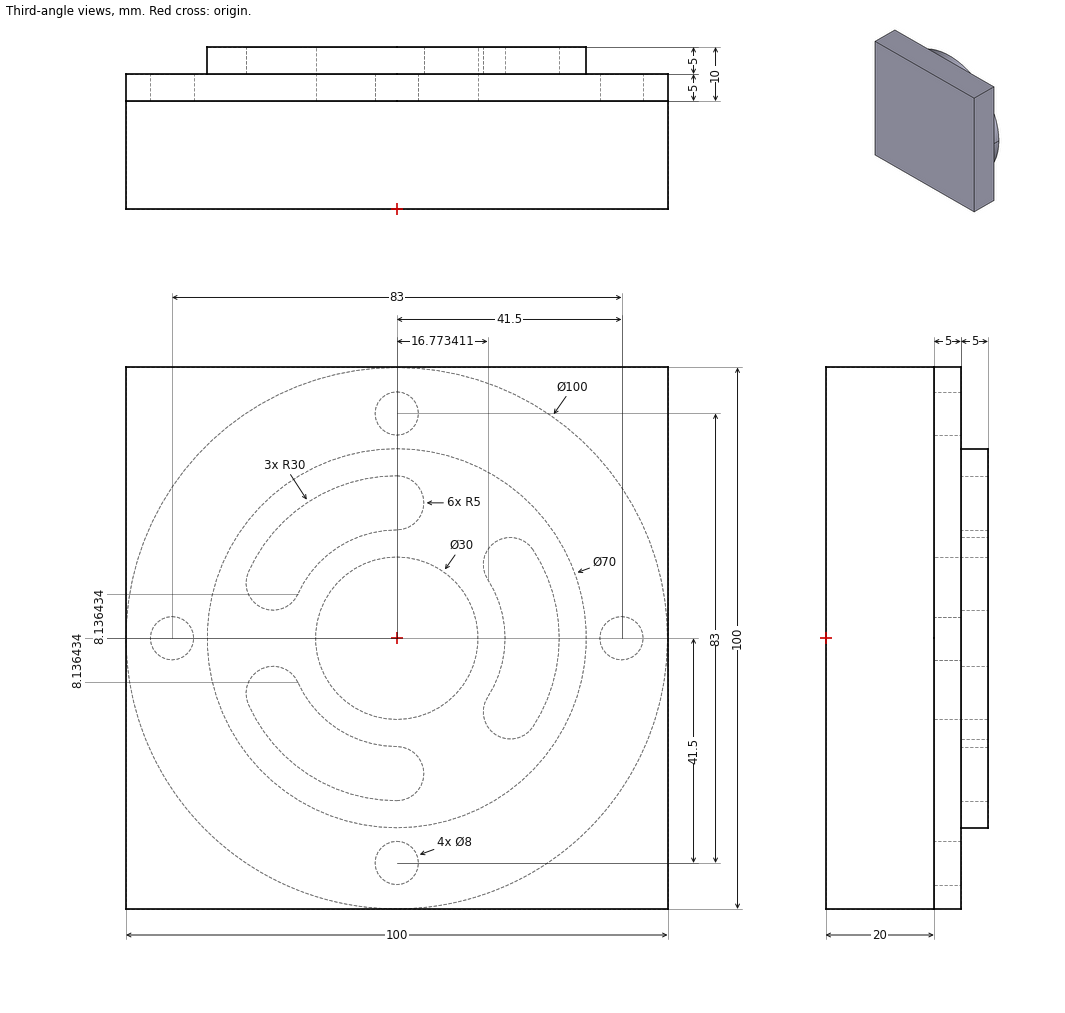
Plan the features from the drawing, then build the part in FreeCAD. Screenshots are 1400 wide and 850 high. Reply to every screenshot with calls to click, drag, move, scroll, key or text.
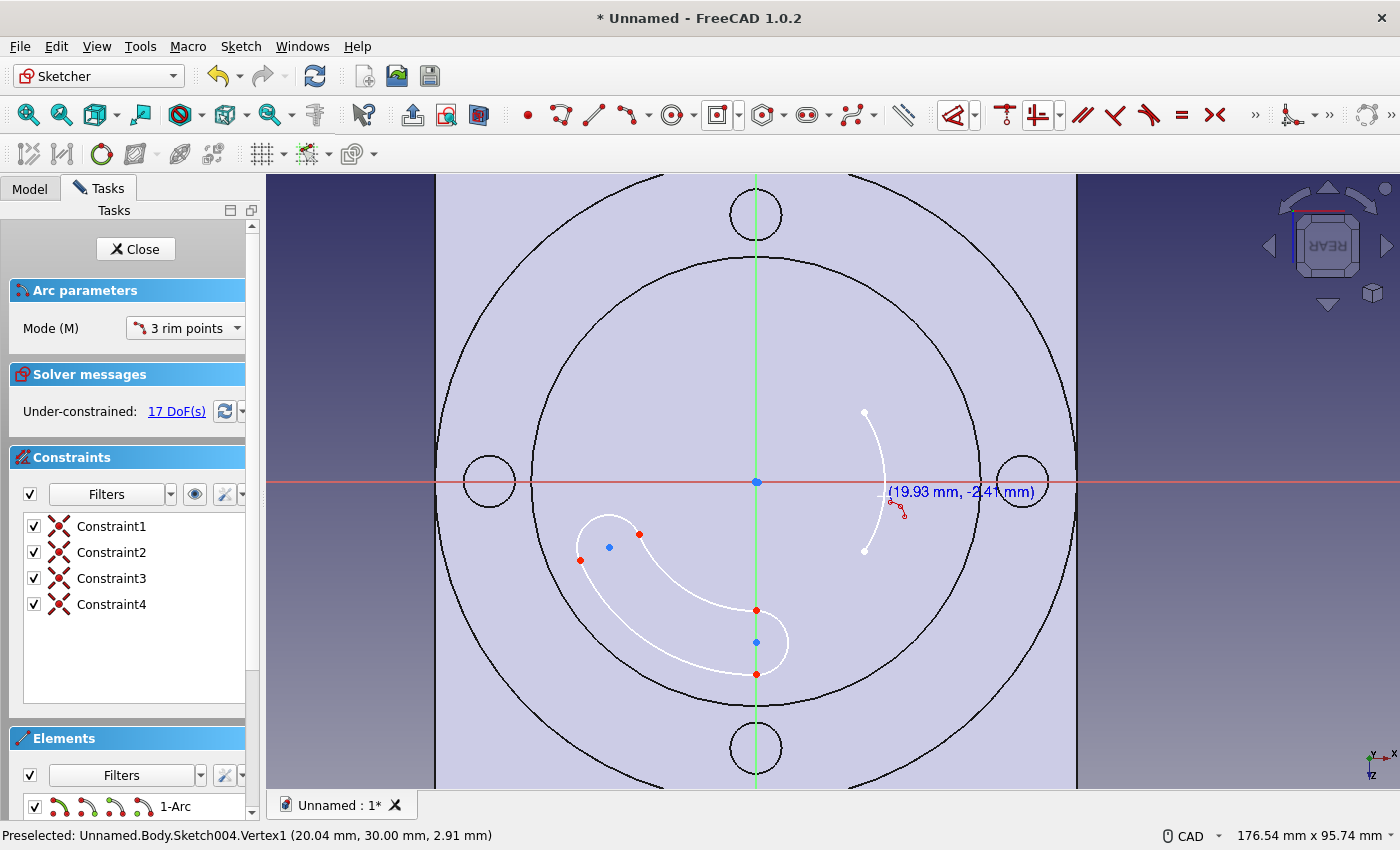
click(864, 552)
click(918, 586)
click(873, 596)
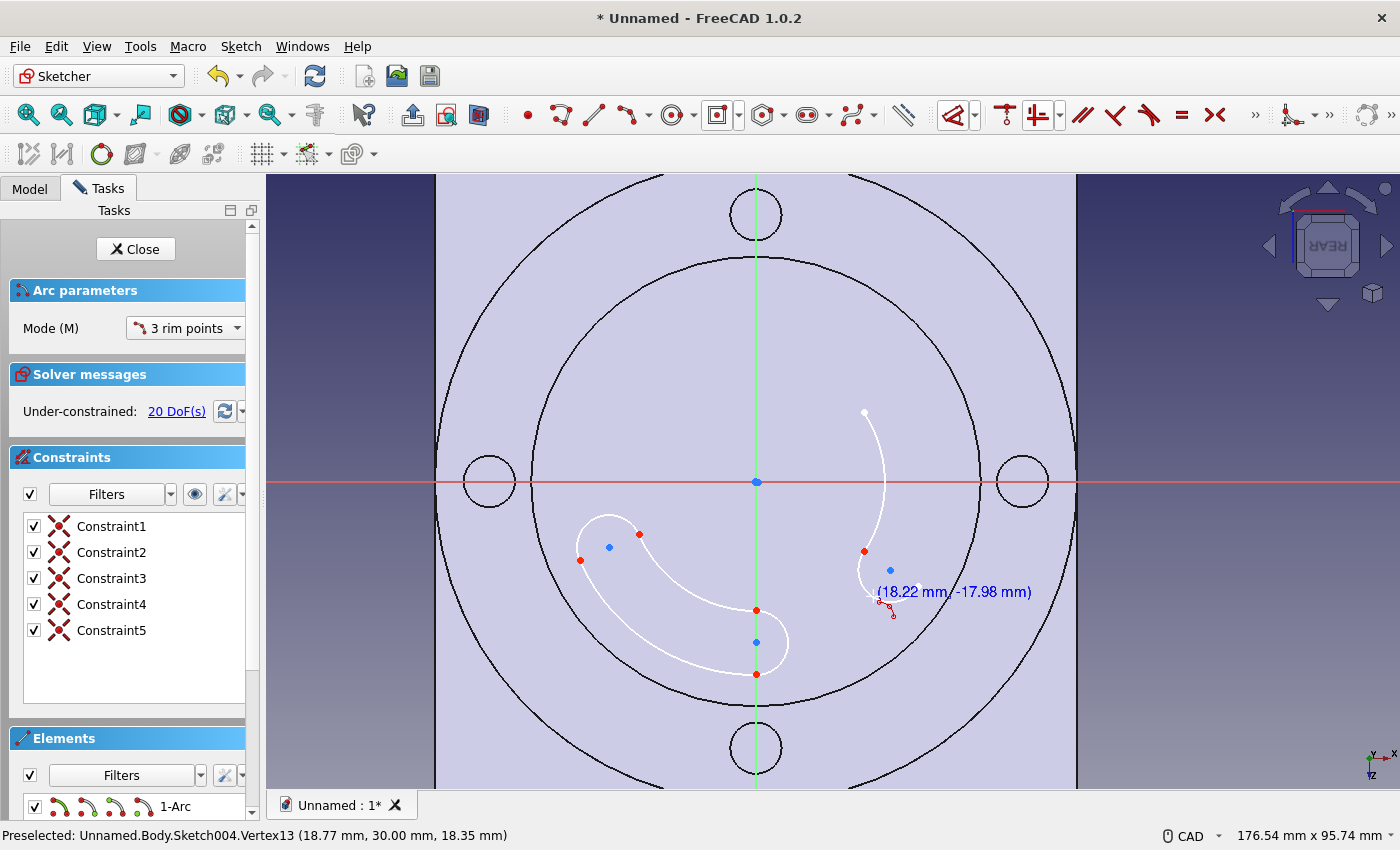
click(918, 587)
click(918, 377)
click(947, 504)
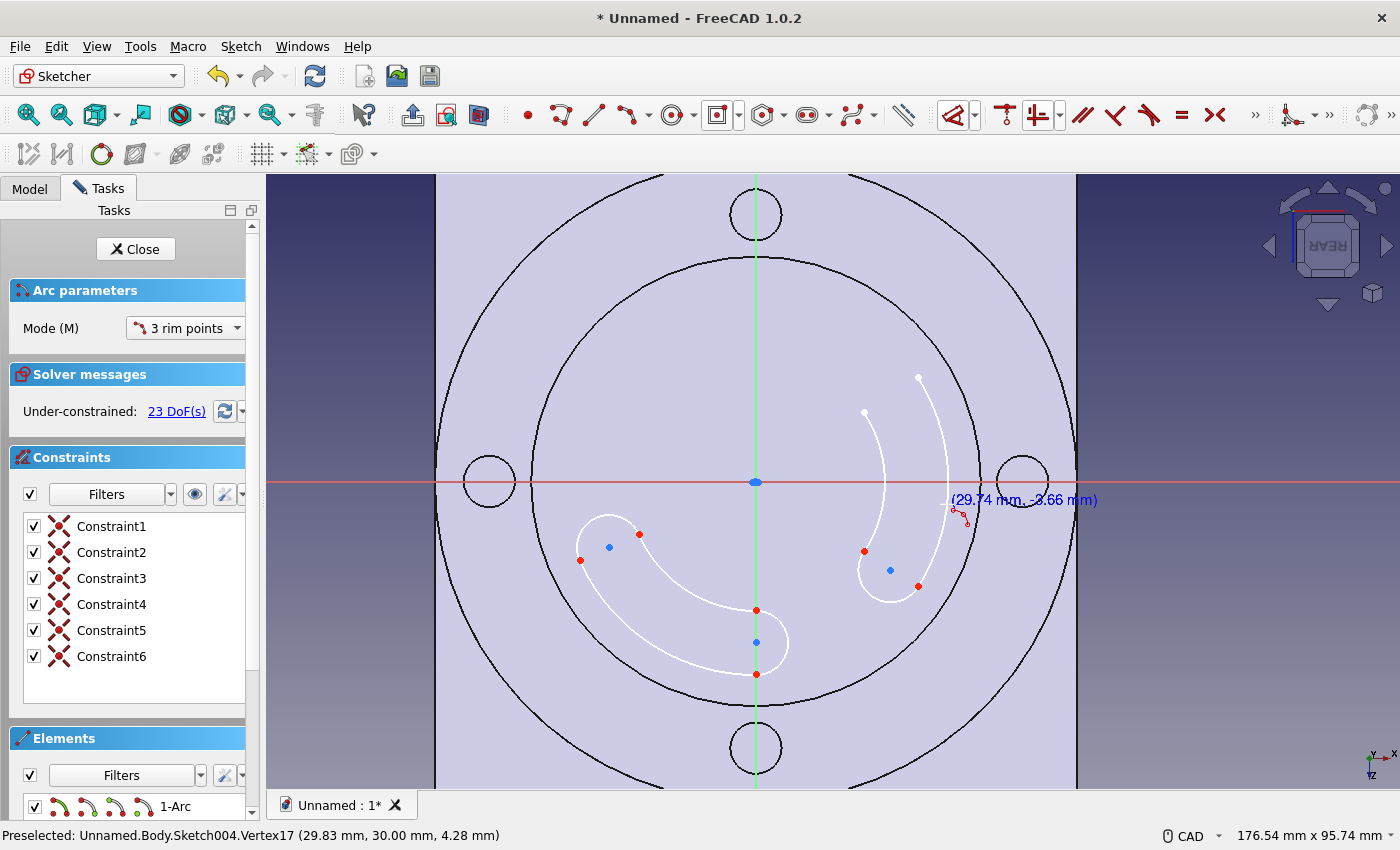
click(918, 378)
click(864, 413)
click(873, 367)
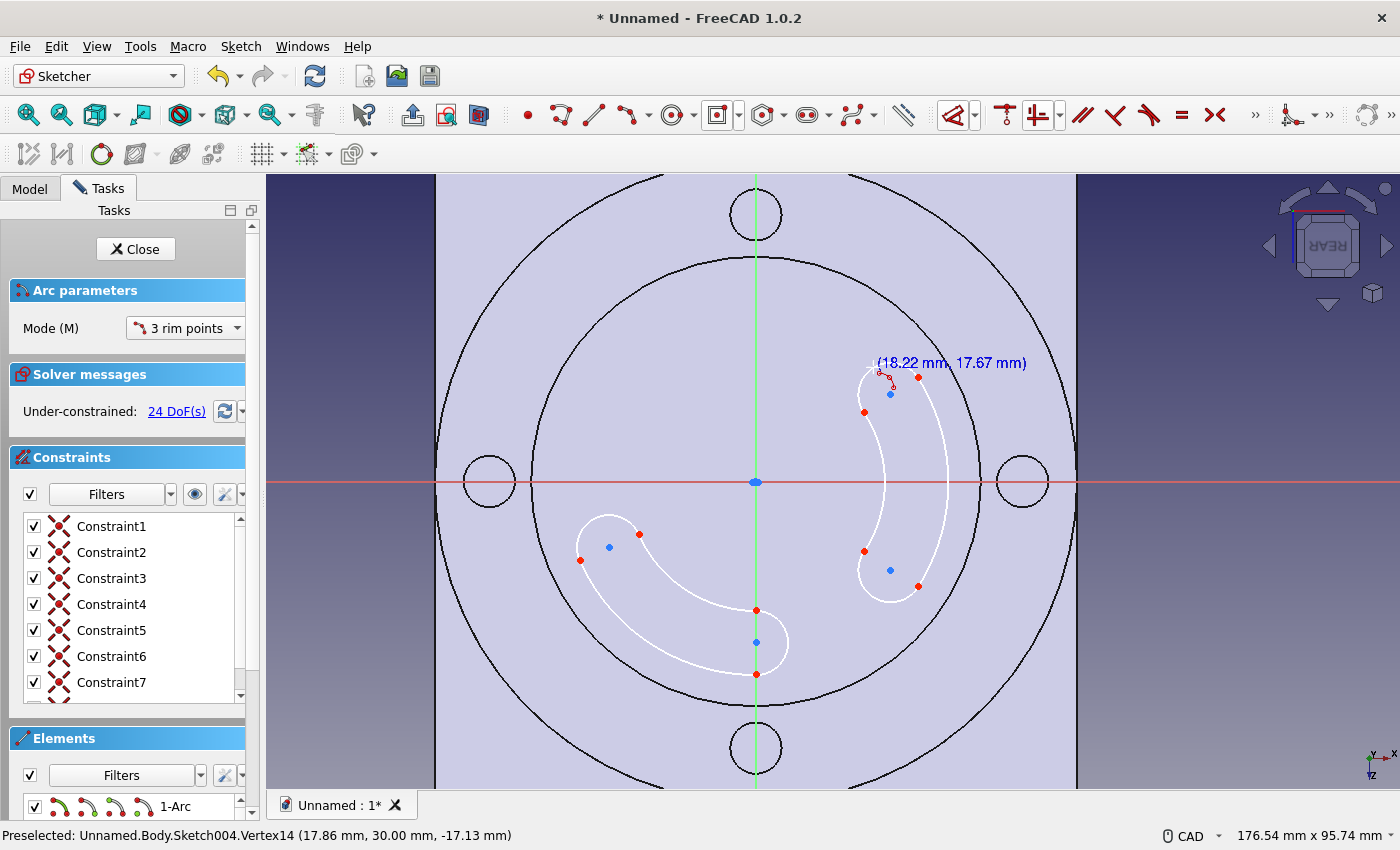
click(639, 429)
click(756, 353)
click(686, 374)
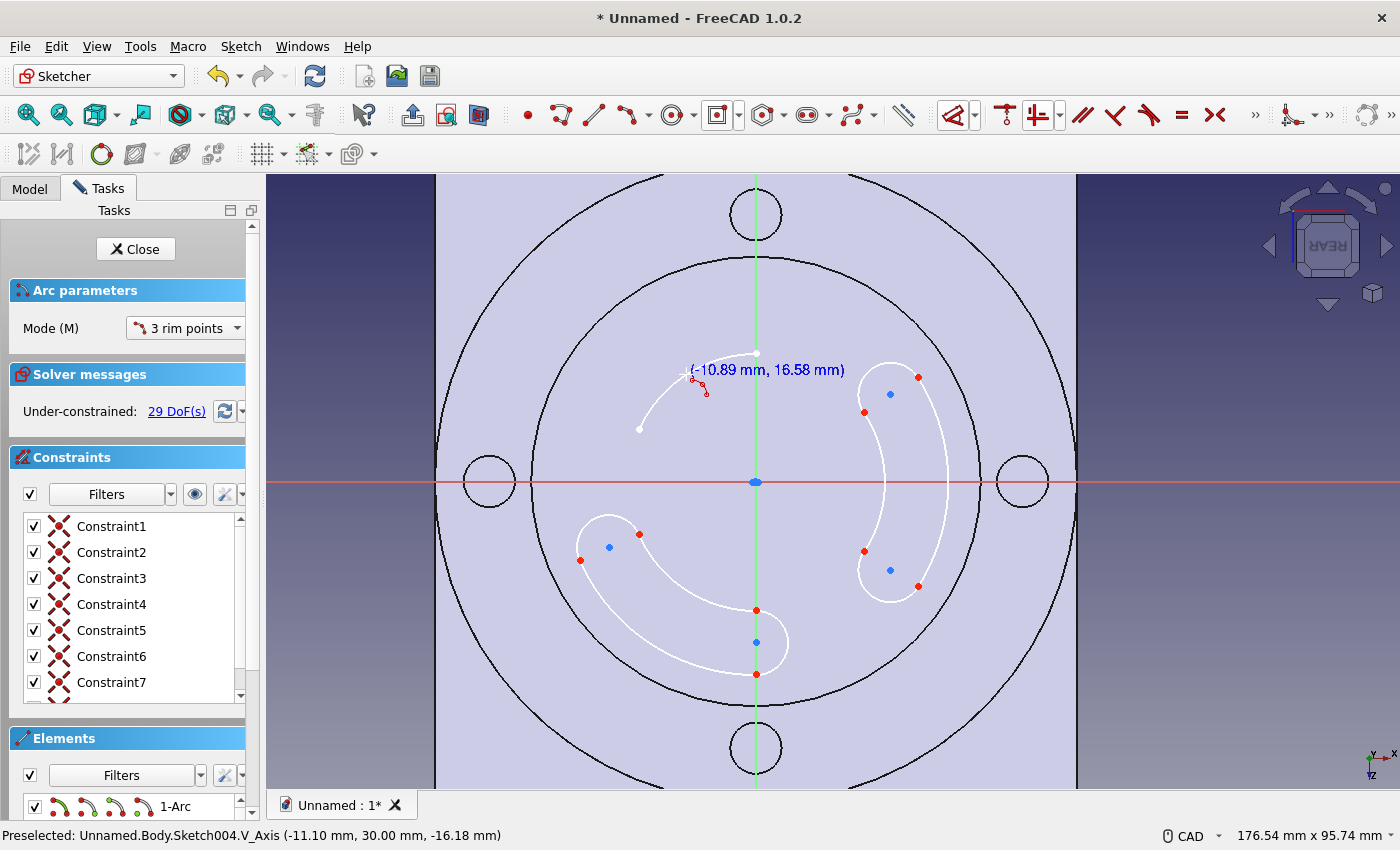
click(756, 354)
click(756, 289)
click(788, 321)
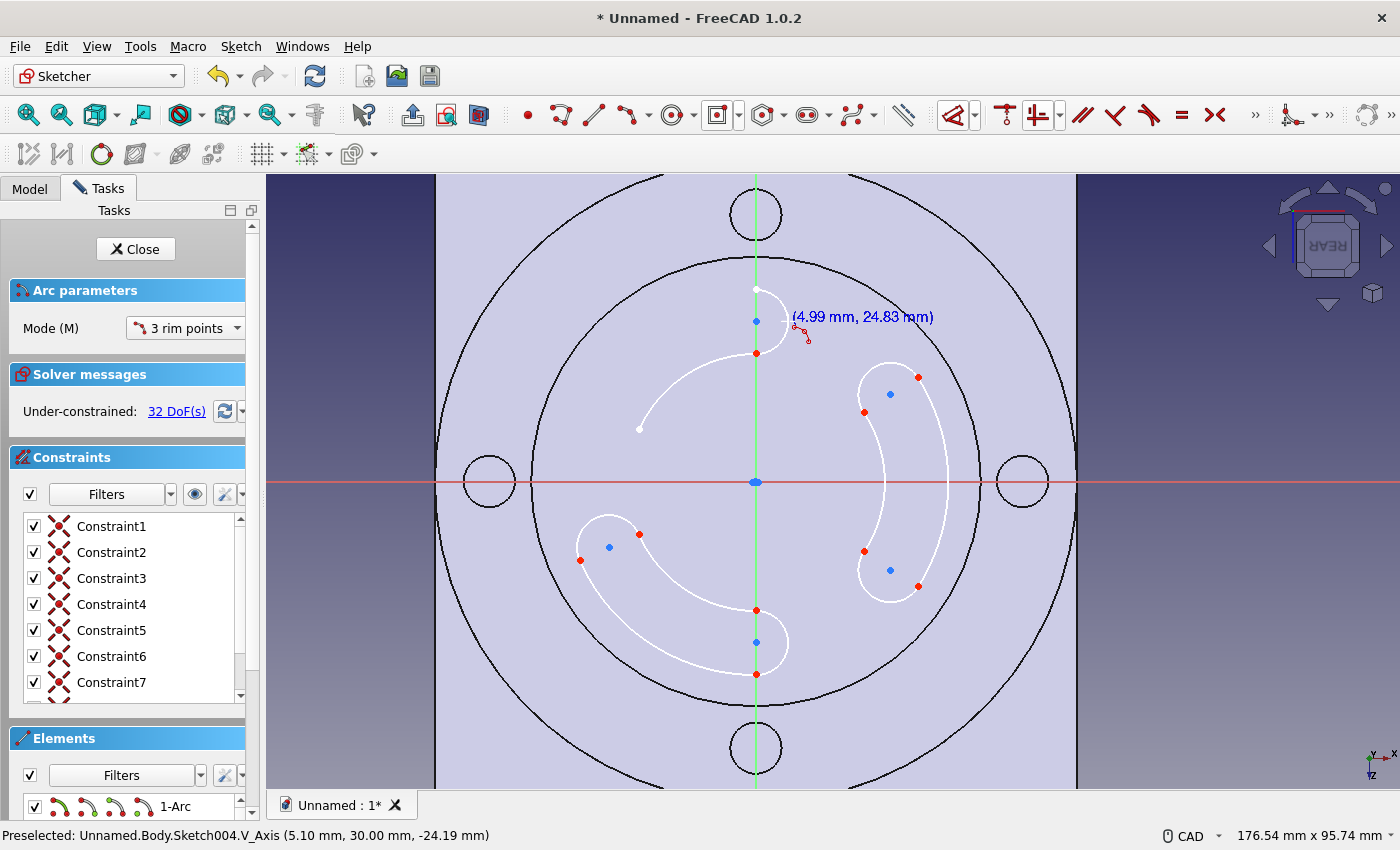
click(756, 290)
click(580, 403)
click(651, 320)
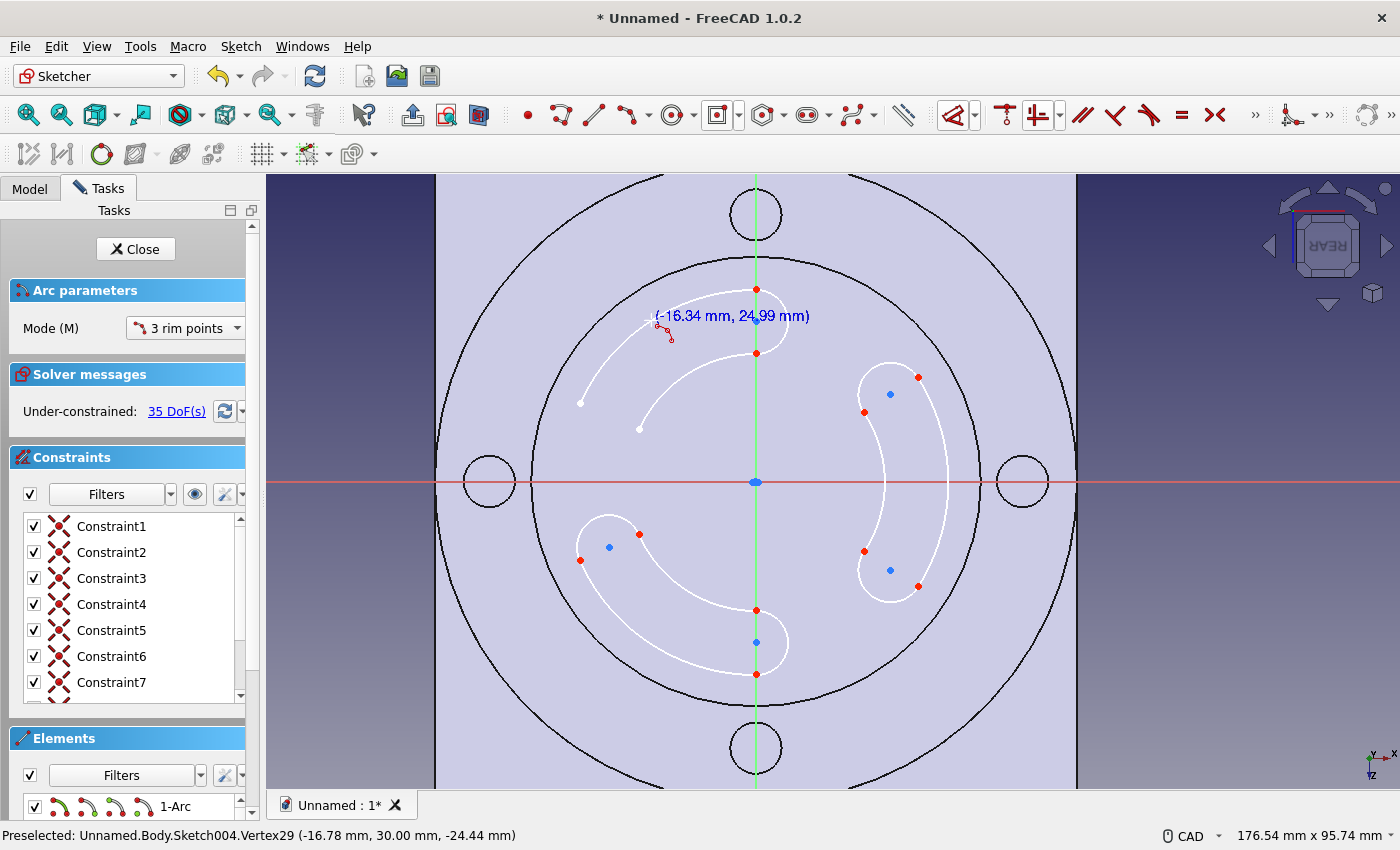
click(580, 404)
click(639, 430)
click(596, 446)
key(Escape)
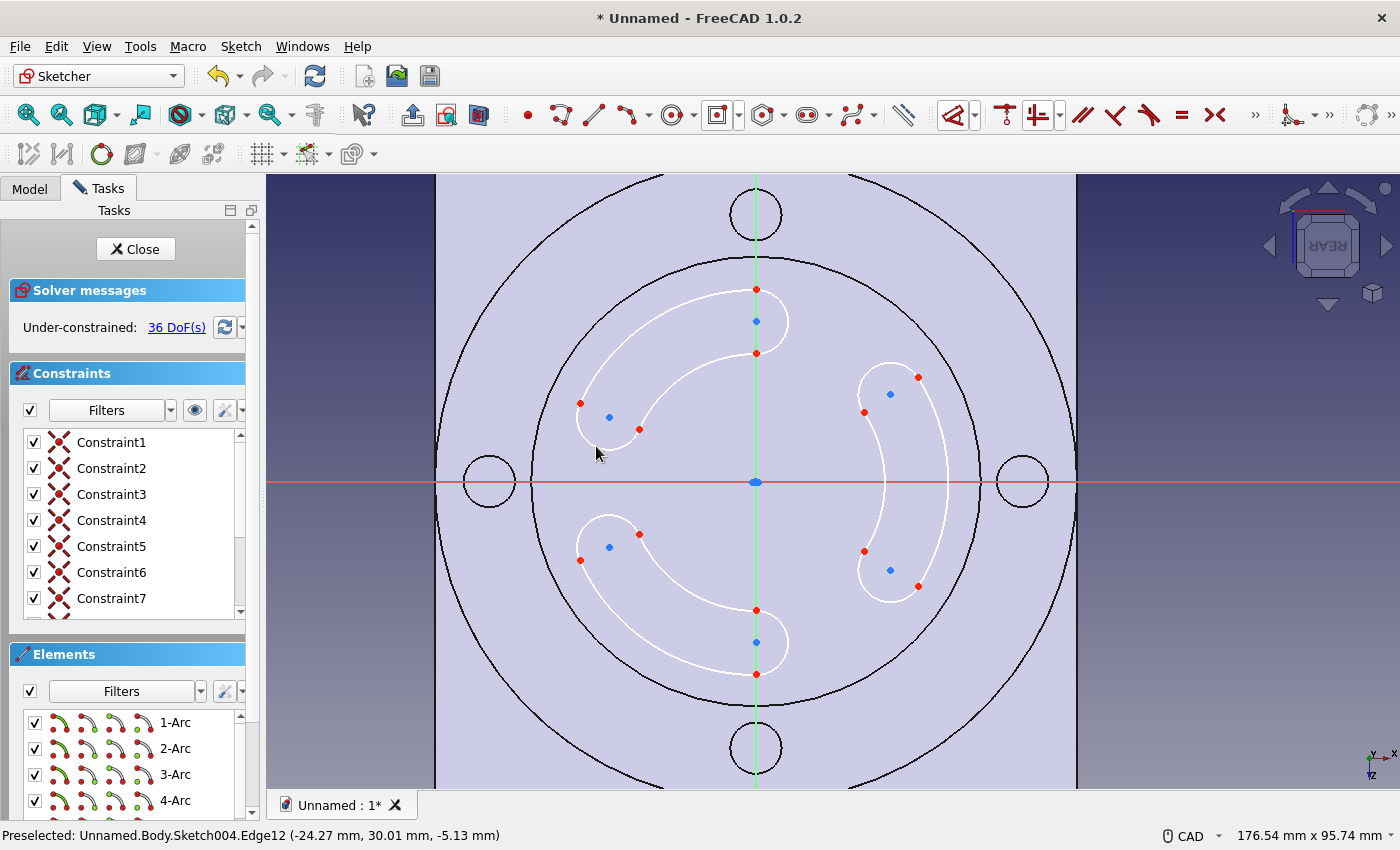
click(616, 516)